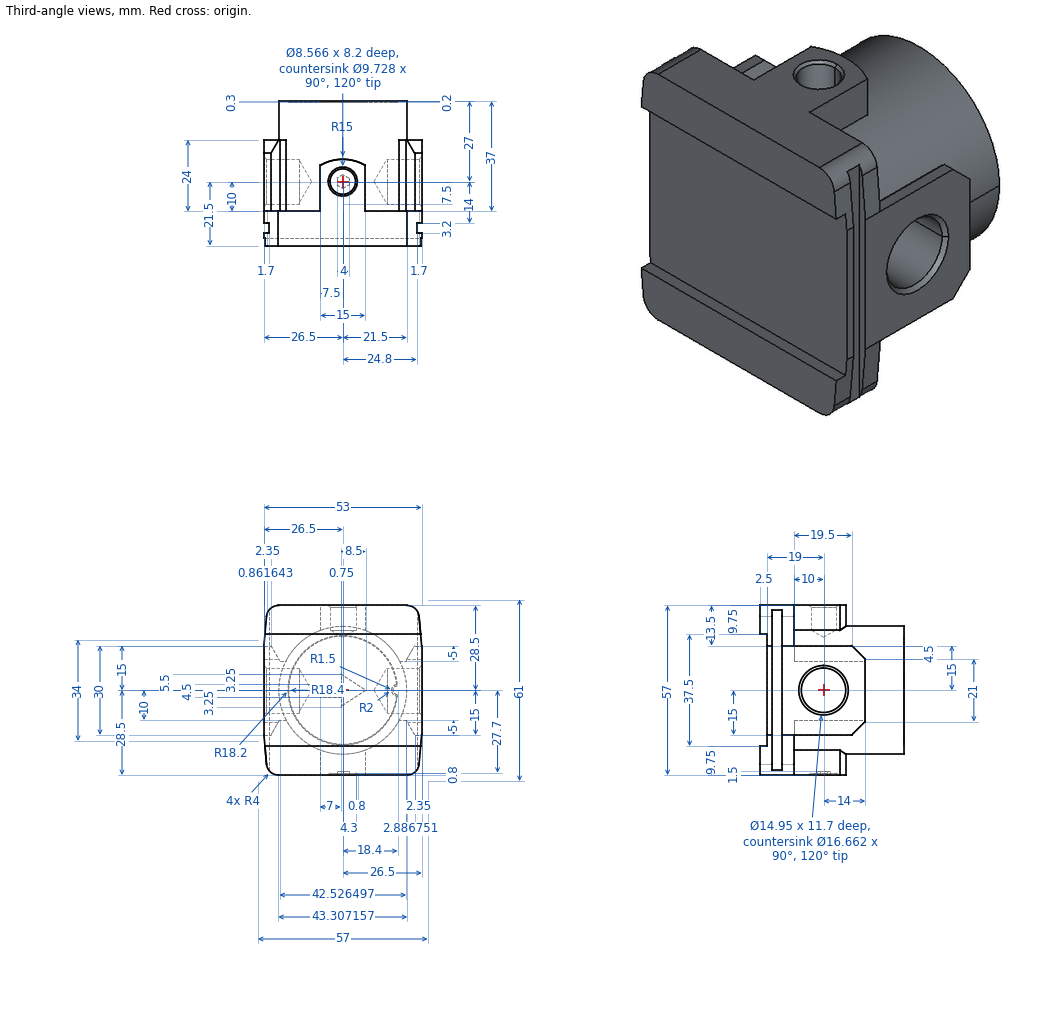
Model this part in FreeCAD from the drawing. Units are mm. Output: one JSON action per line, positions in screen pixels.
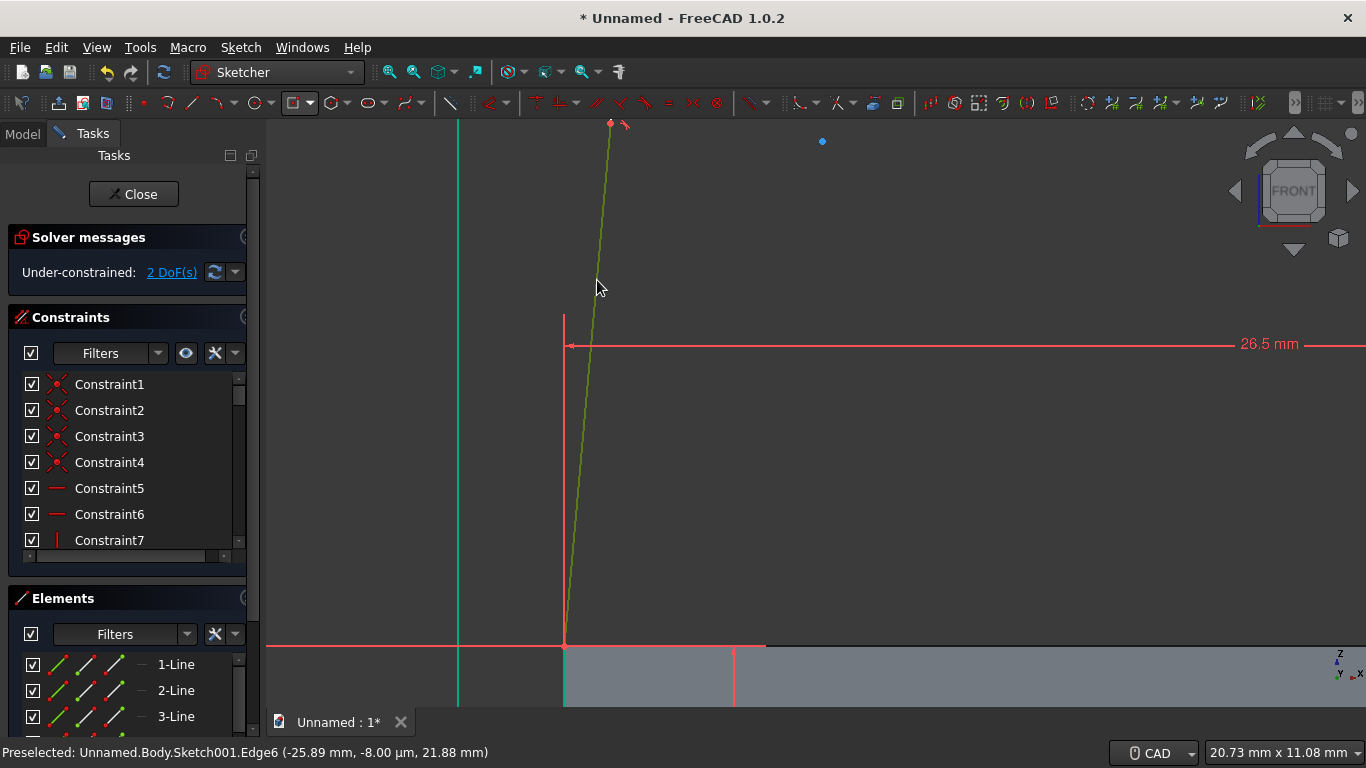
{"action": "left_click", "coordinate": [508, 104]}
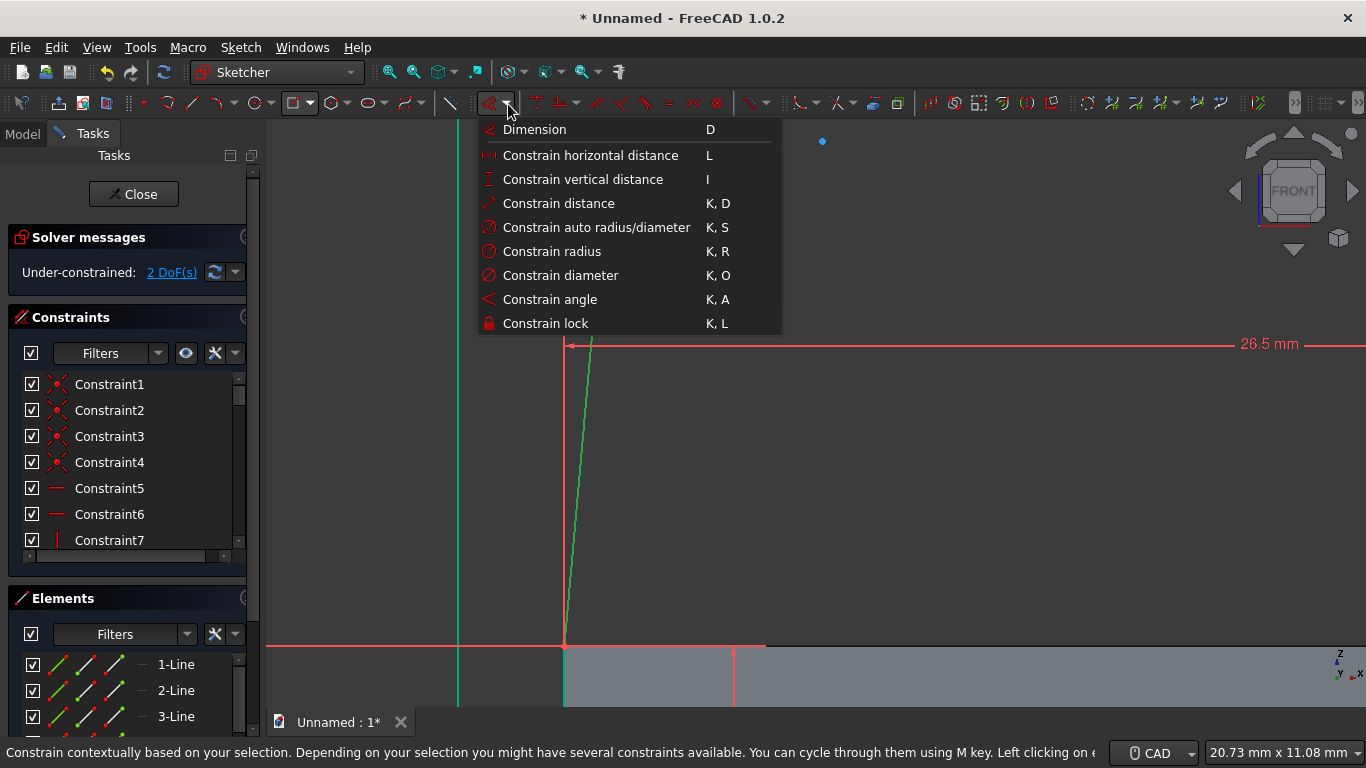
{"action": "left_click", "coordinate": [630, 155]}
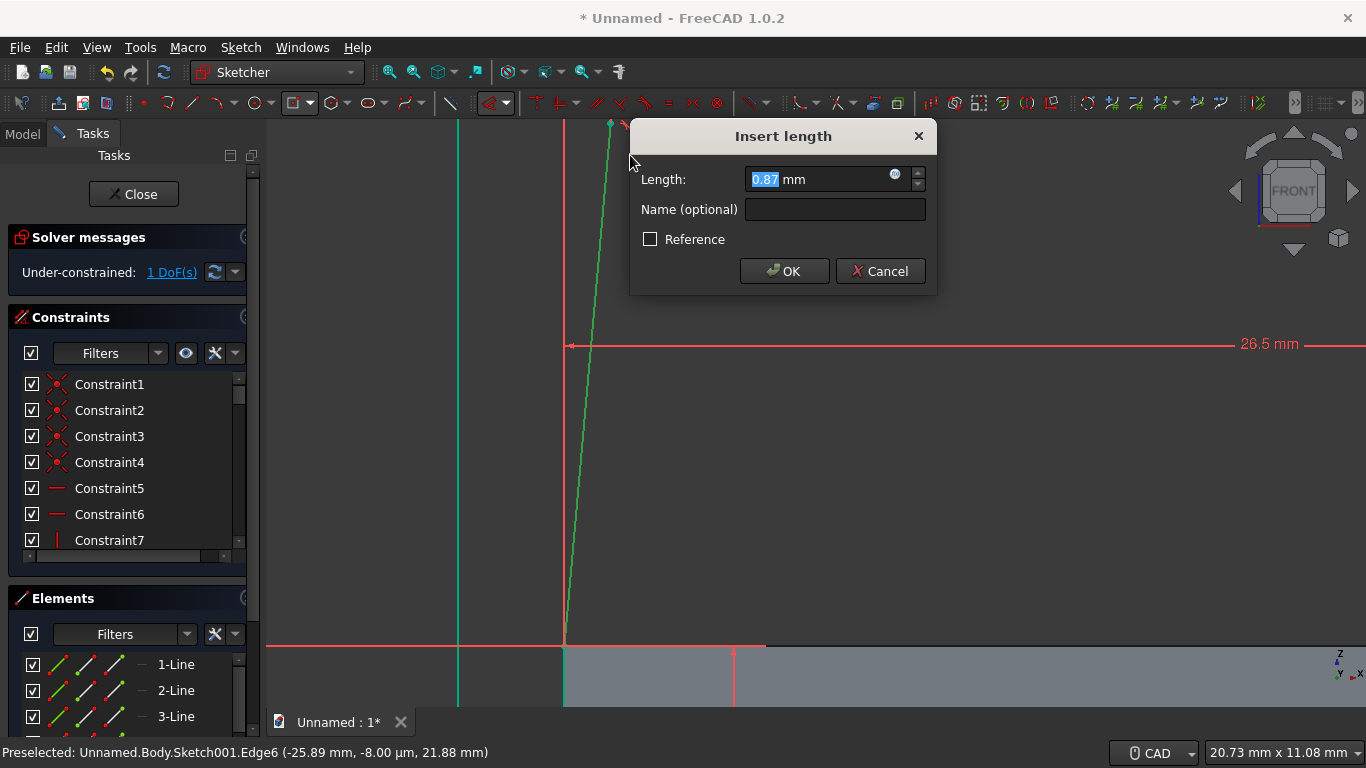
{"action": "type", "text": "0.861643"}
{"action": "key", "text": "Return"}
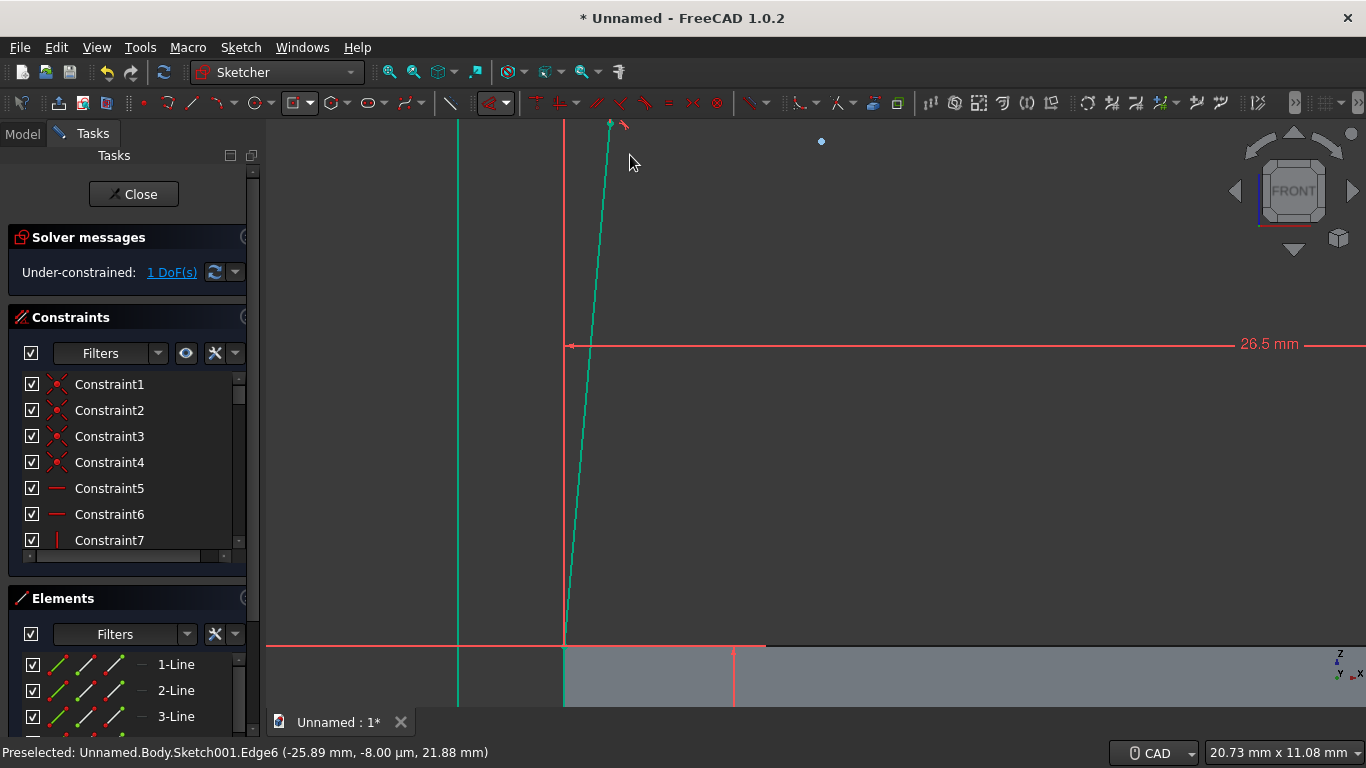
{"action": "scroll", "coordinate": [595, 285], "scroll_direction": "down", "scroll_amount": 11}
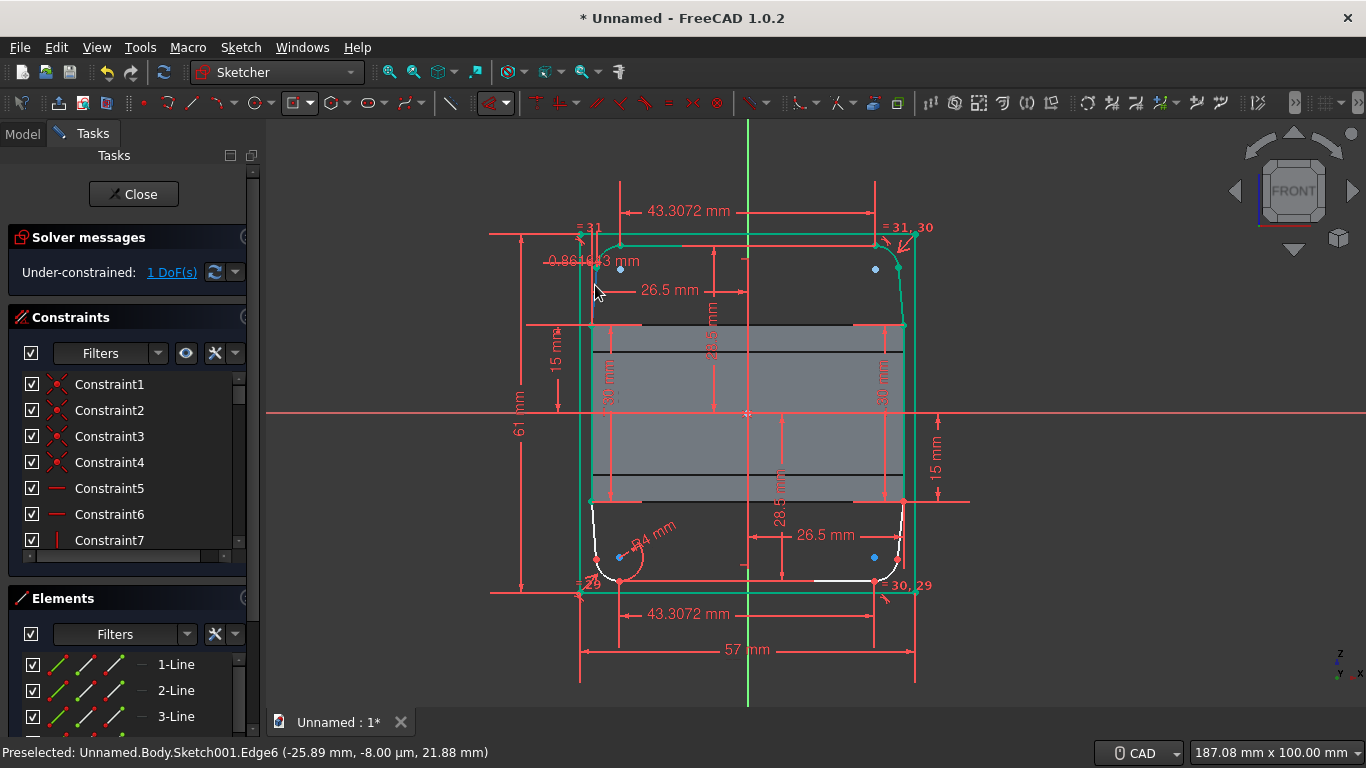
{"action": "scroll", "coordinate": [593, 519], "scroll_direction": "up", "scroll_amount": 11}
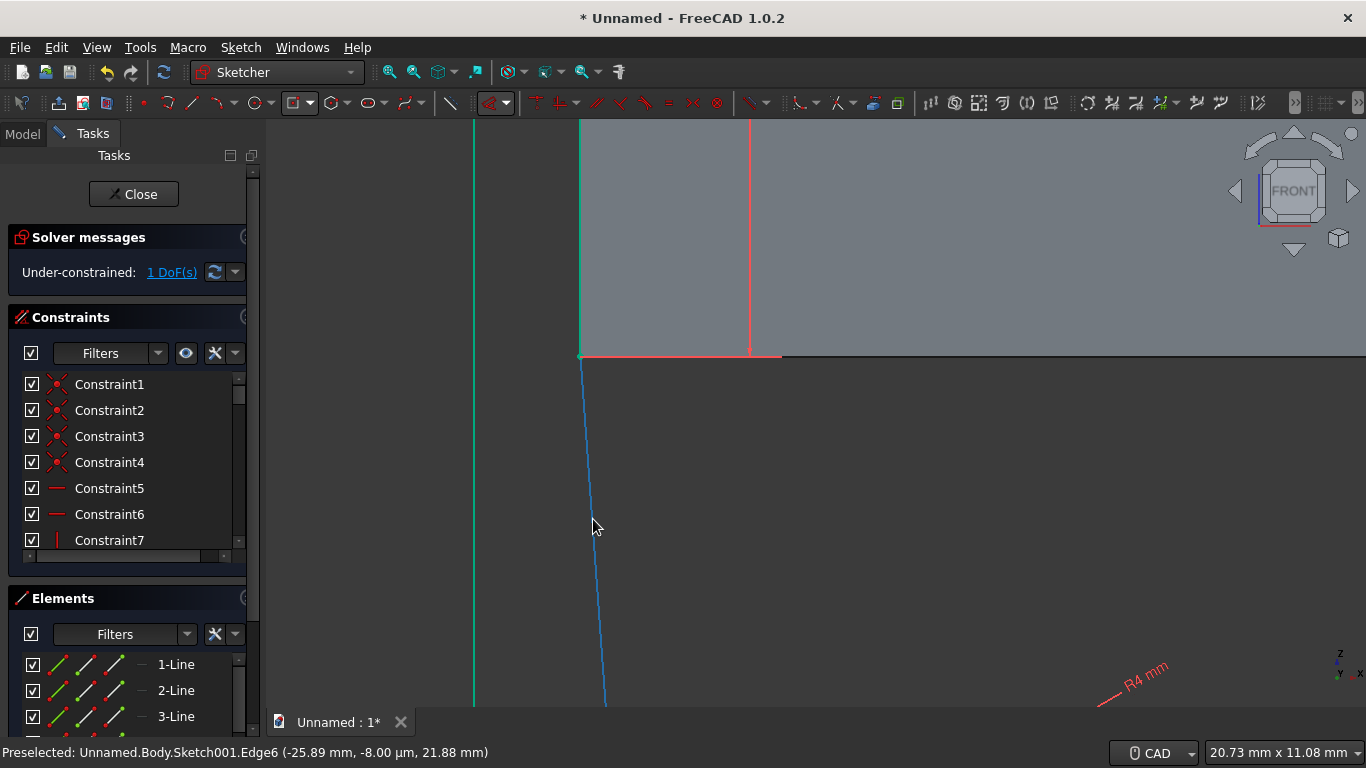
{"action": "left_click", "coordinate": [592, 513]}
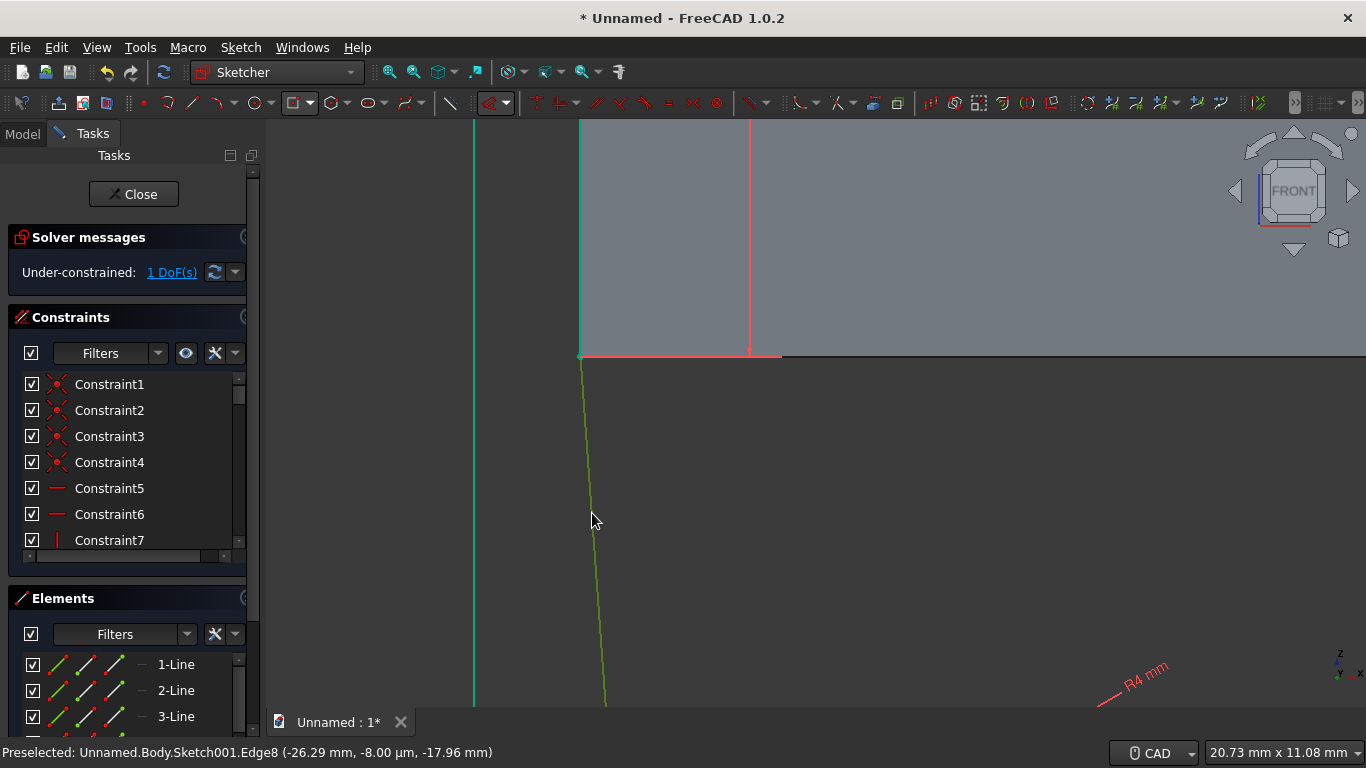
{"action": "left_click", "coordinate": [508, 104]}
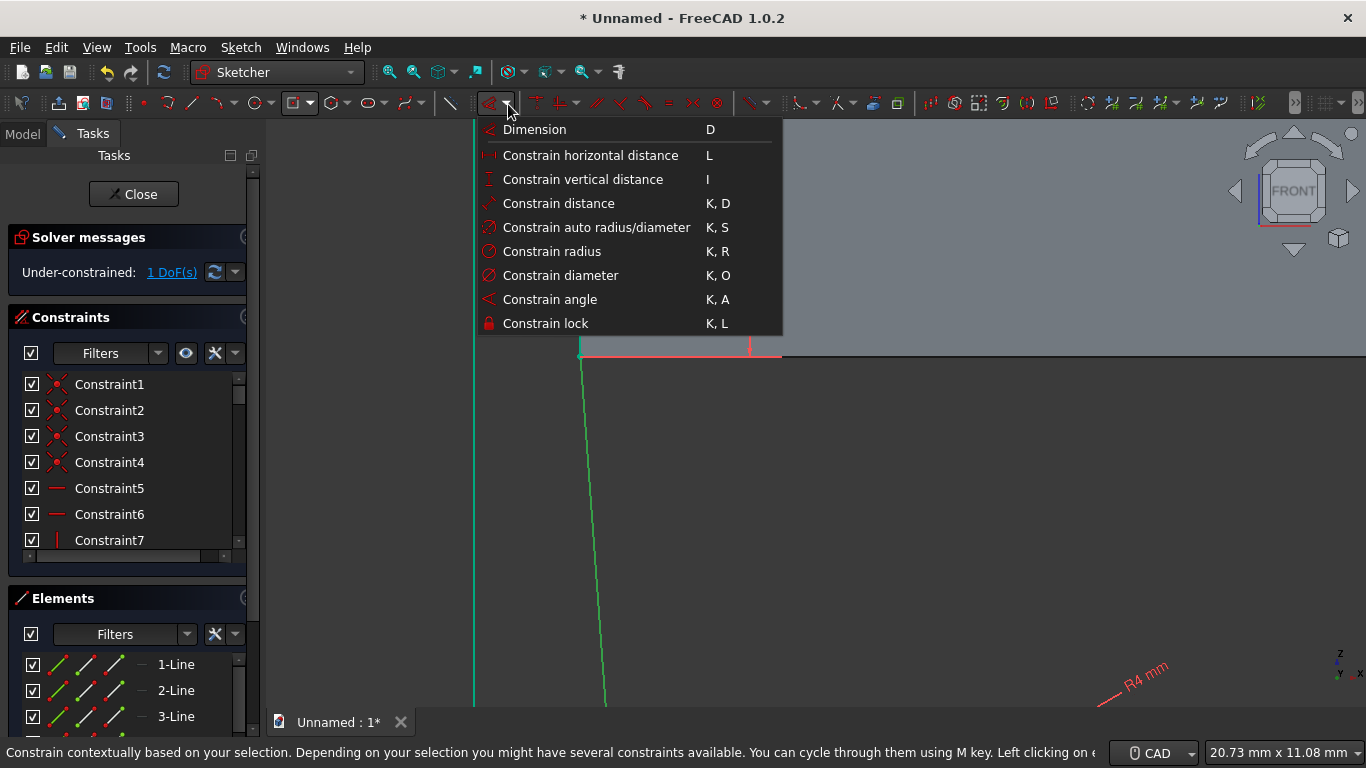
{"action": "left_click", "coordinate": [630, 155]}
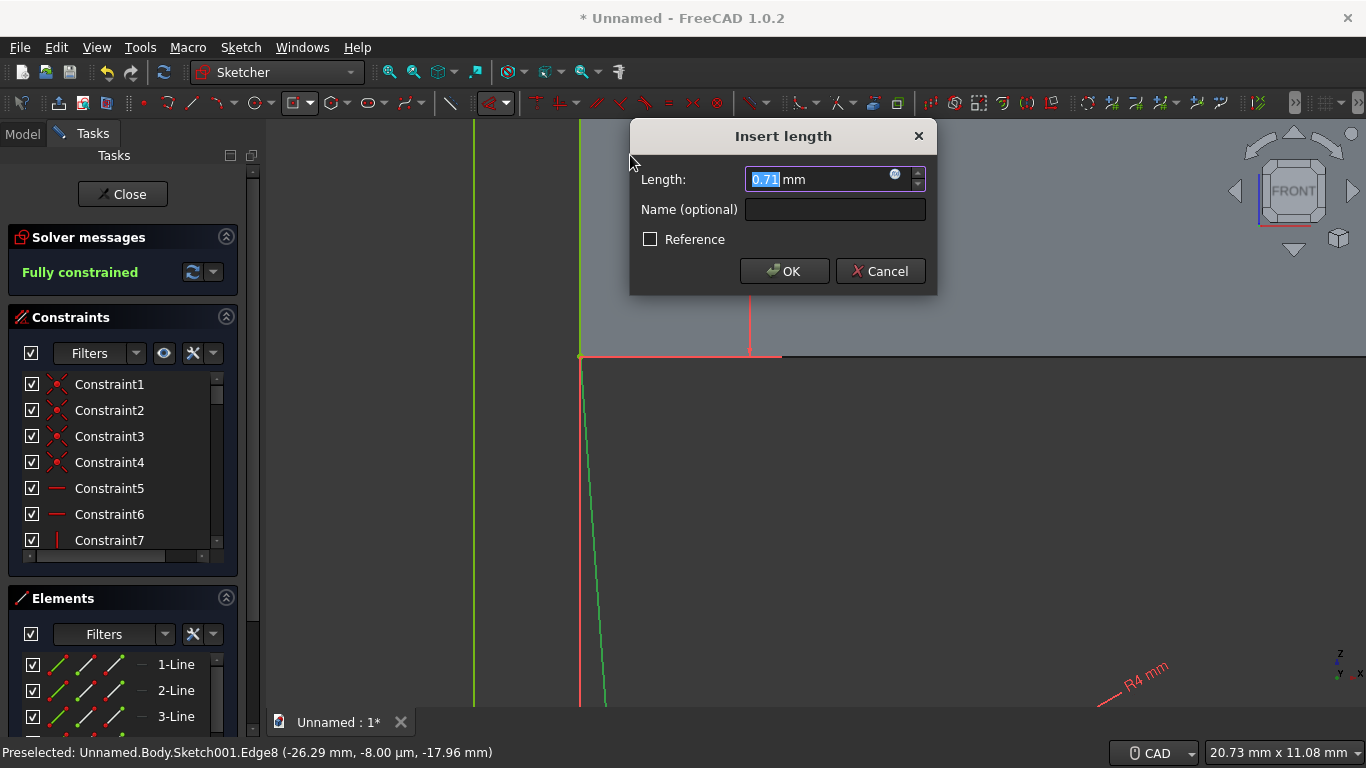
{"action": "type", "text": "0.861643"}
{"action": "key", "text": "Return"}